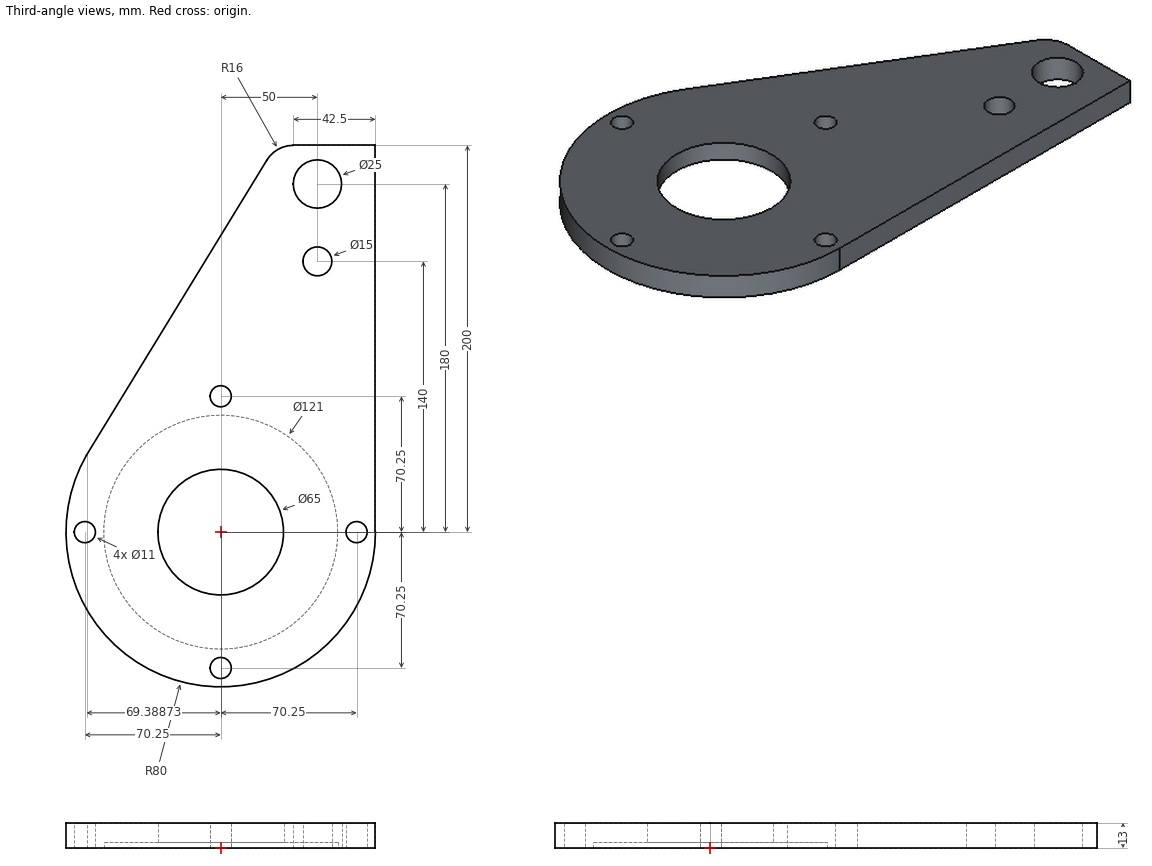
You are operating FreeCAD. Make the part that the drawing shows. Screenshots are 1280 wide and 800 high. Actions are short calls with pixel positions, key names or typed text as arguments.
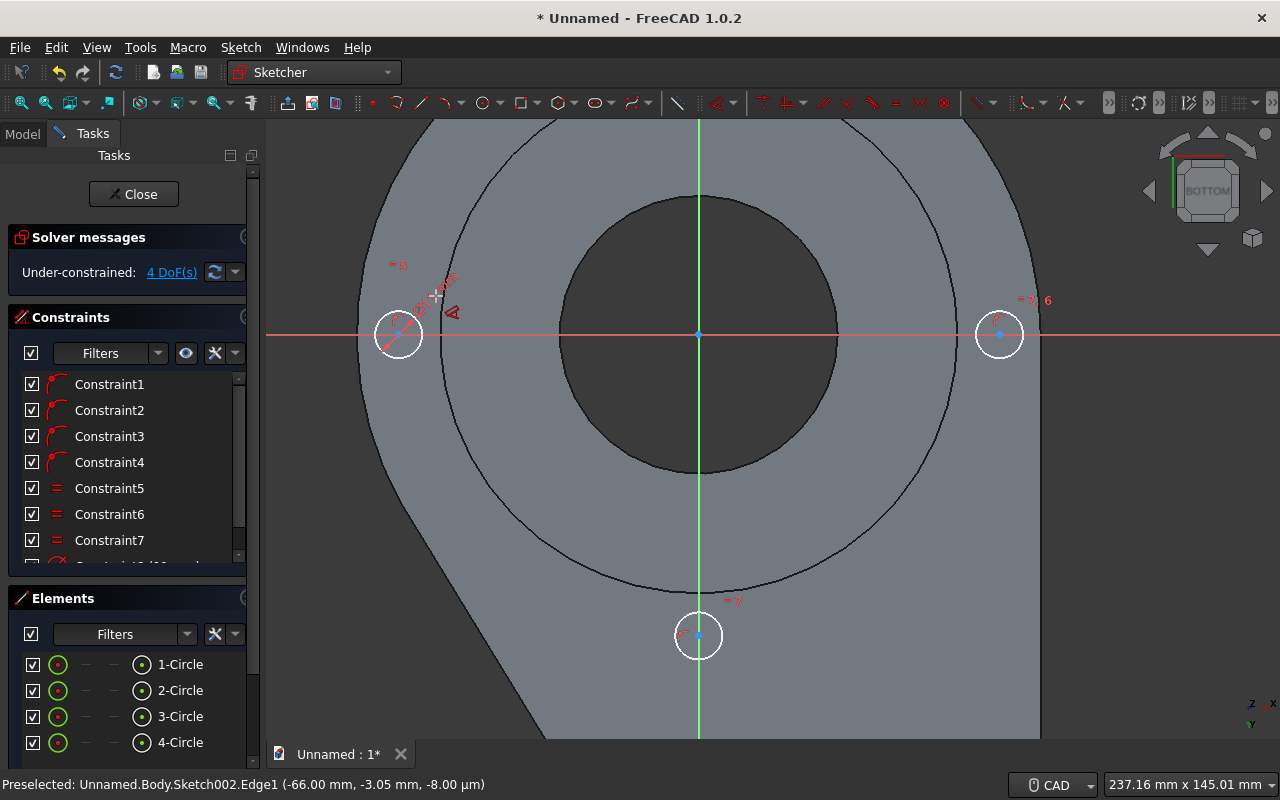
click(399, 335)
click(549, 369)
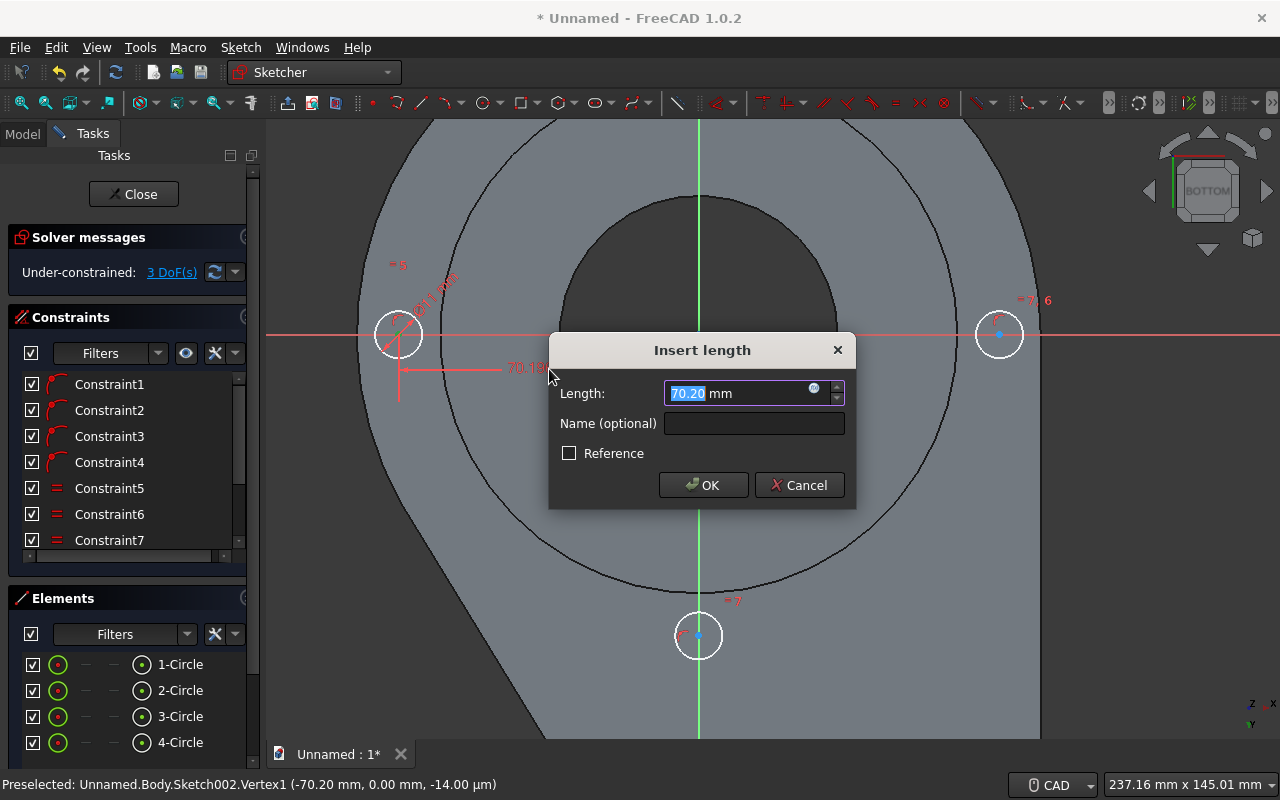
text(70.25)
key(Return)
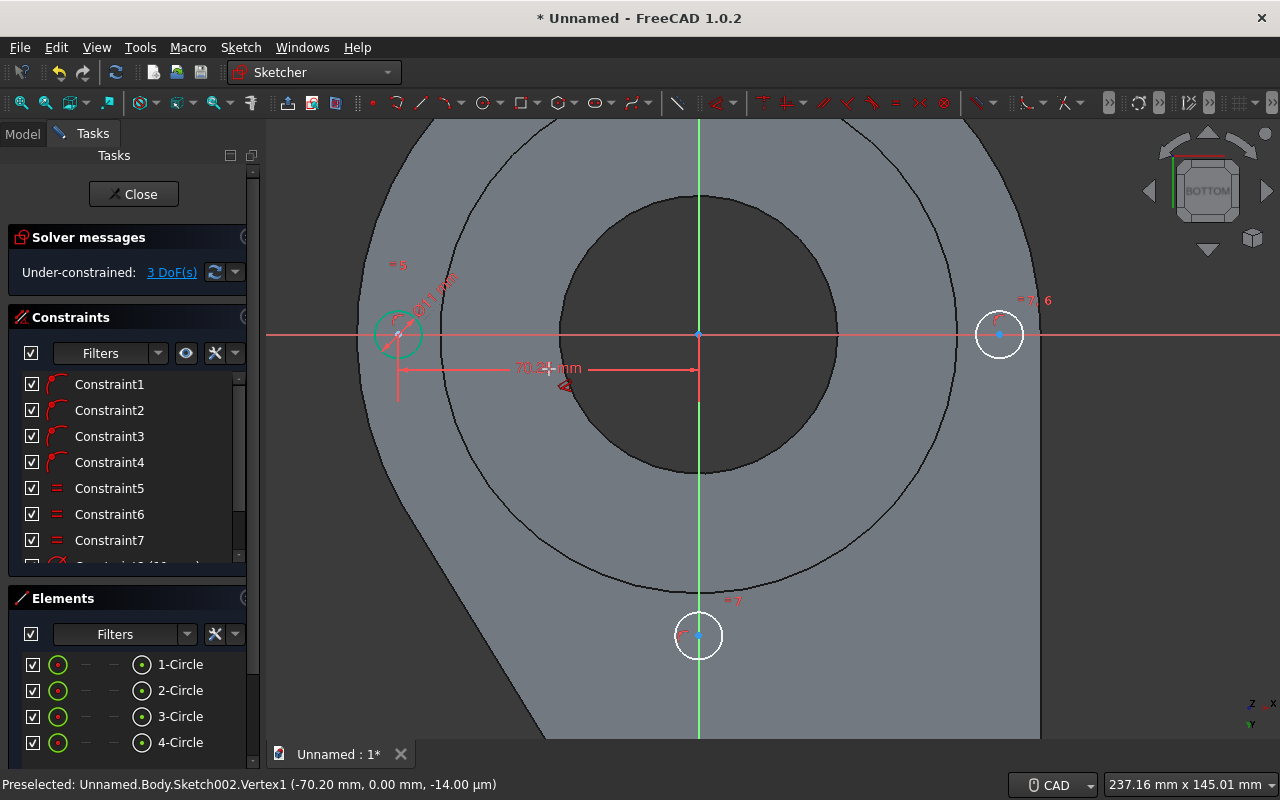
scroll(716, 621, down, 2)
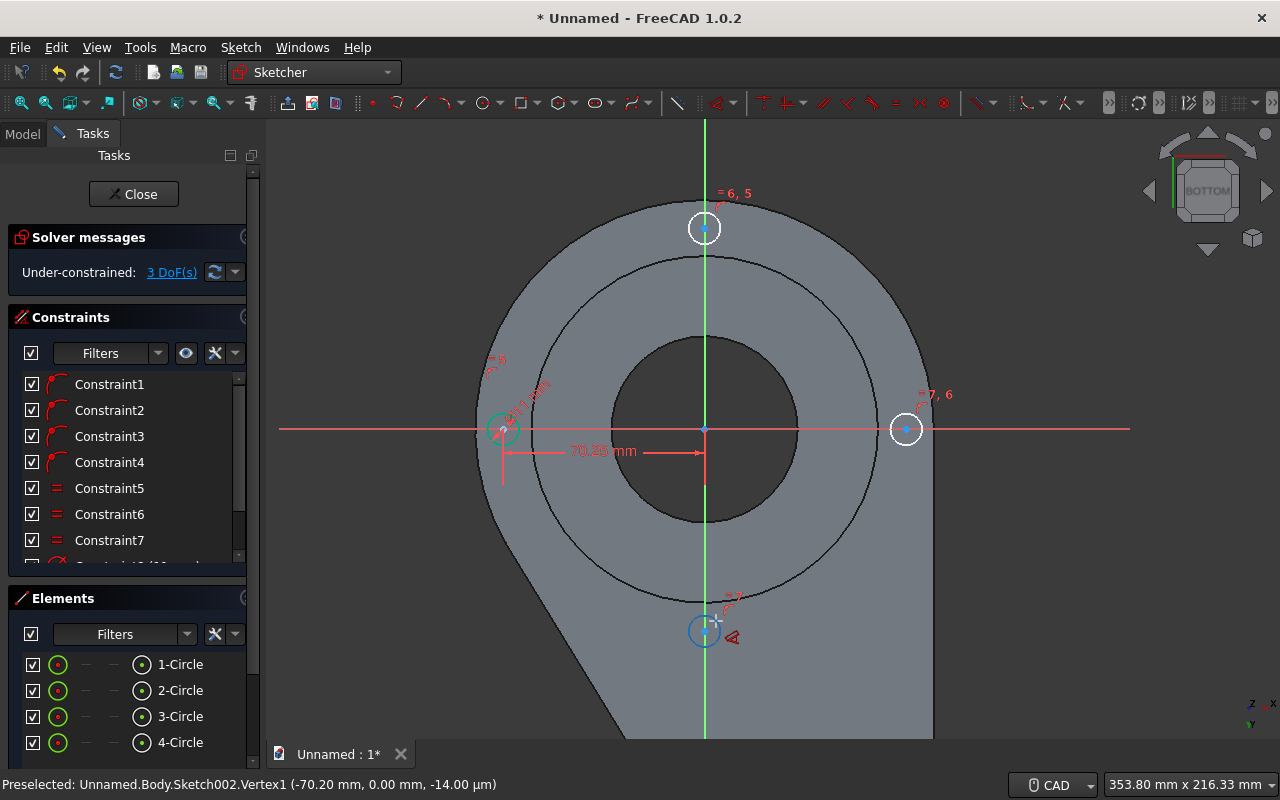
click(705, 228)
click(739, 329)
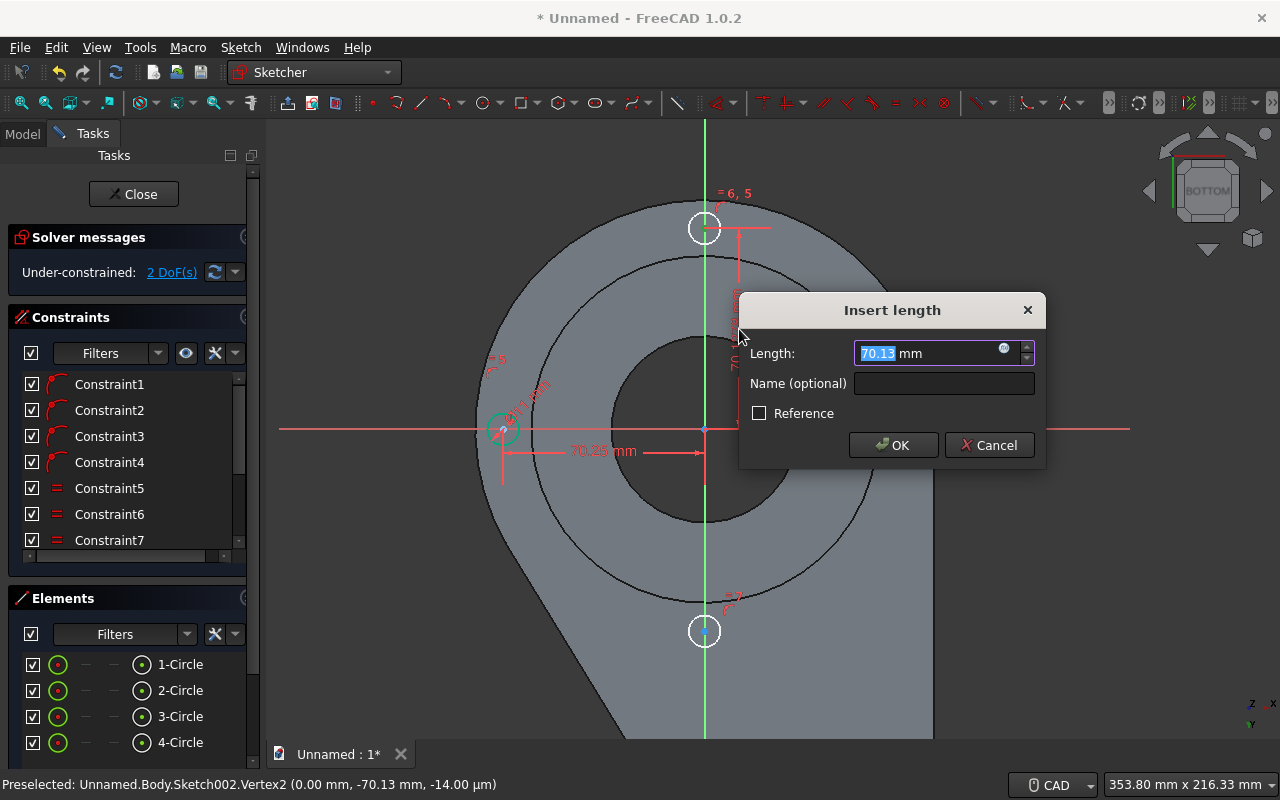
text(70.25)
key(Return)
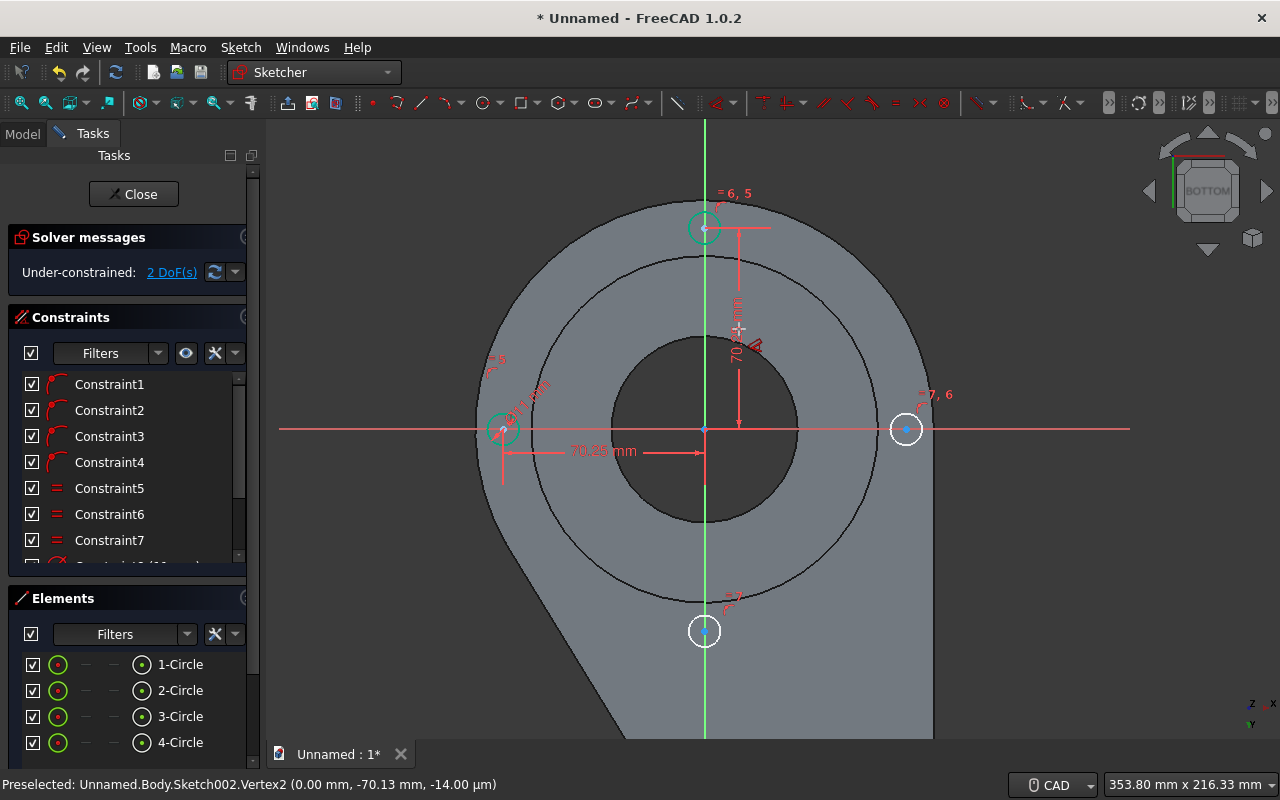
click(906, 429)
click(805, 463)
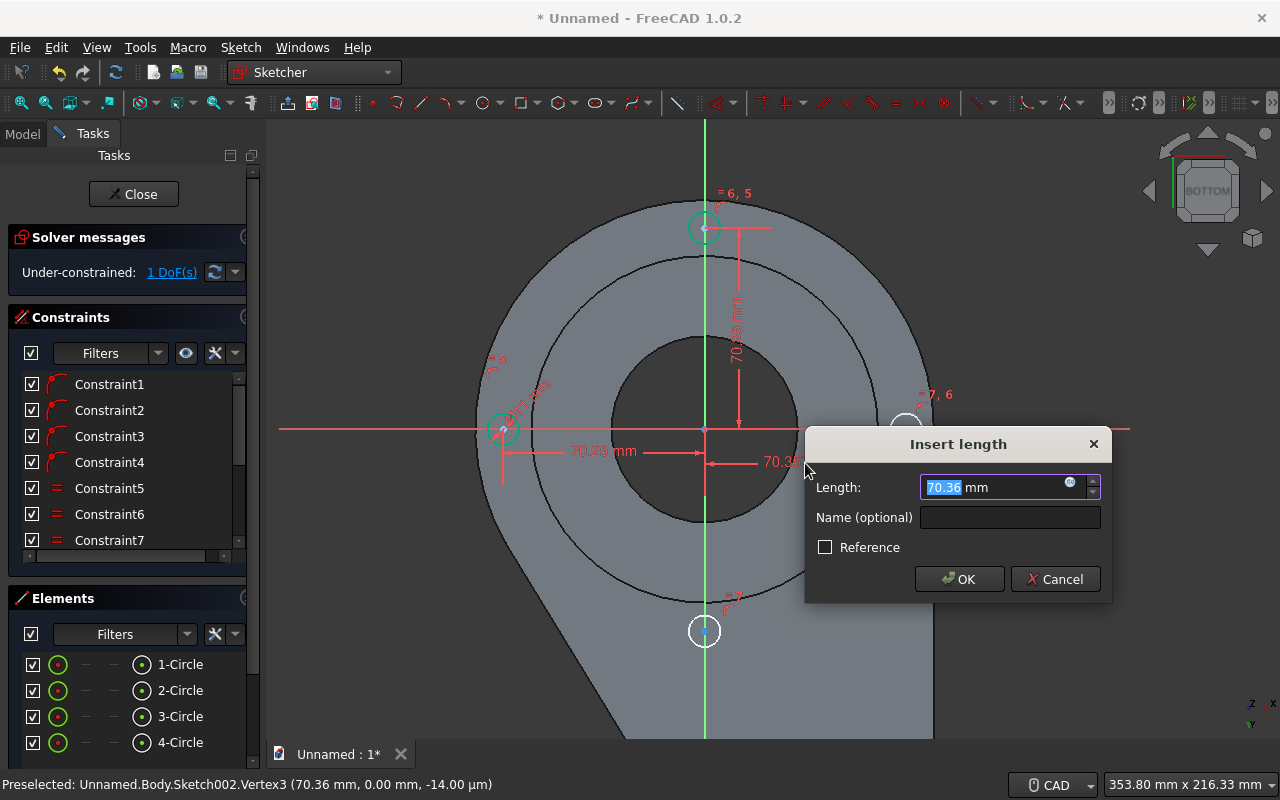
text(70.25)
key(Return)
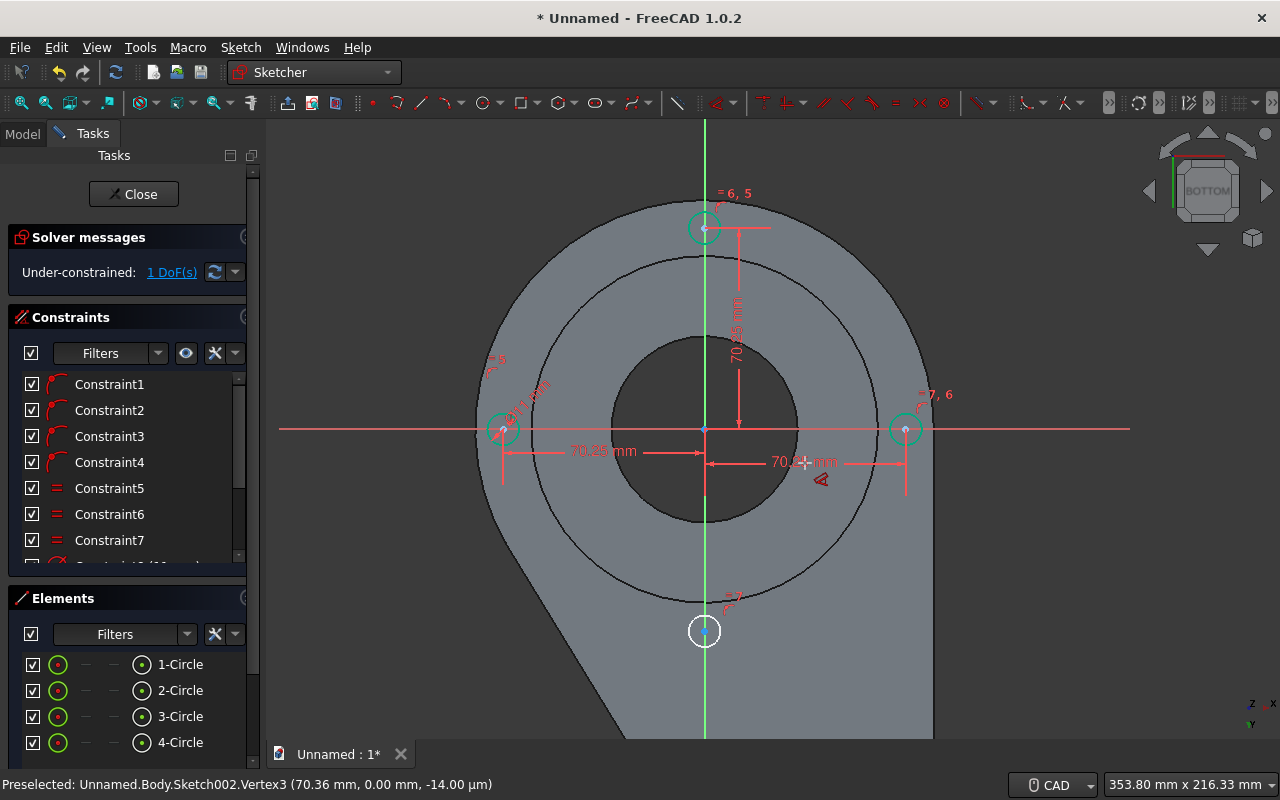
click(705, 631)
click(739, 530)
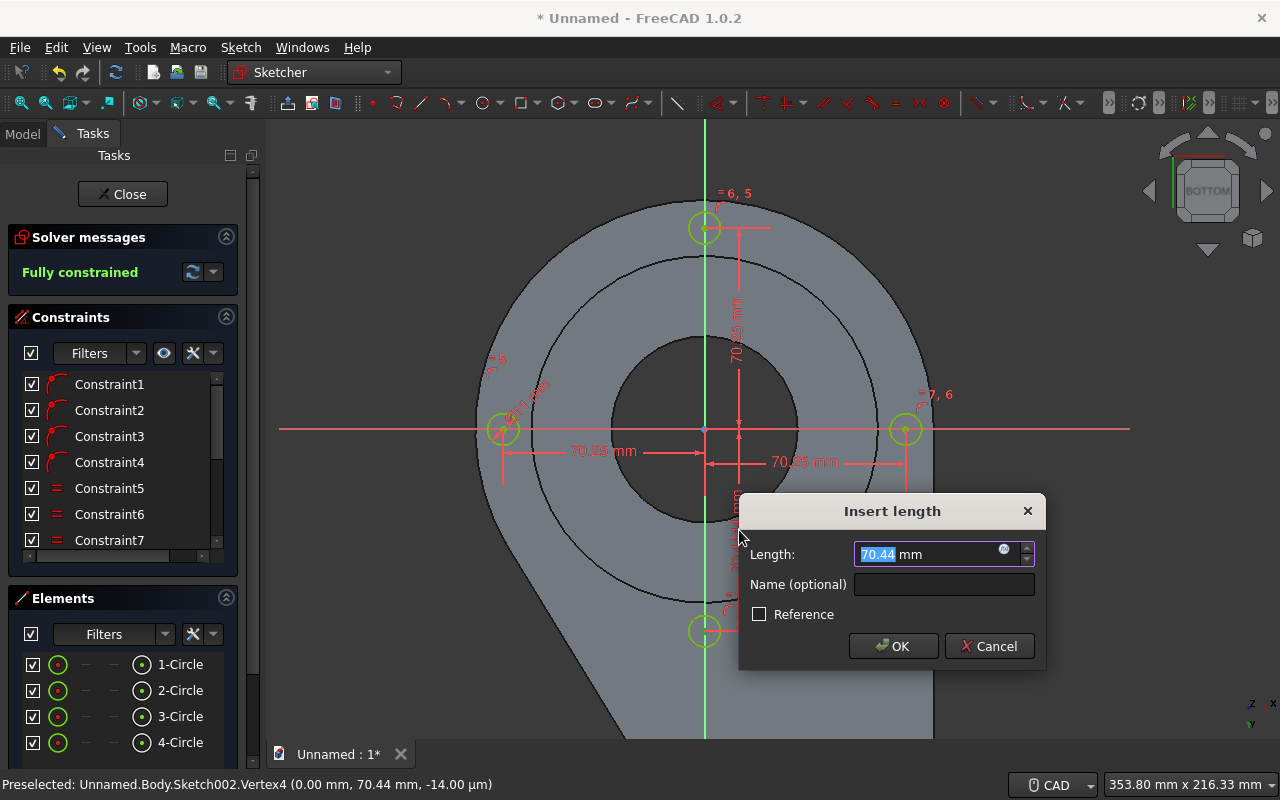
text(70.25)
key(Return)
key(Escape)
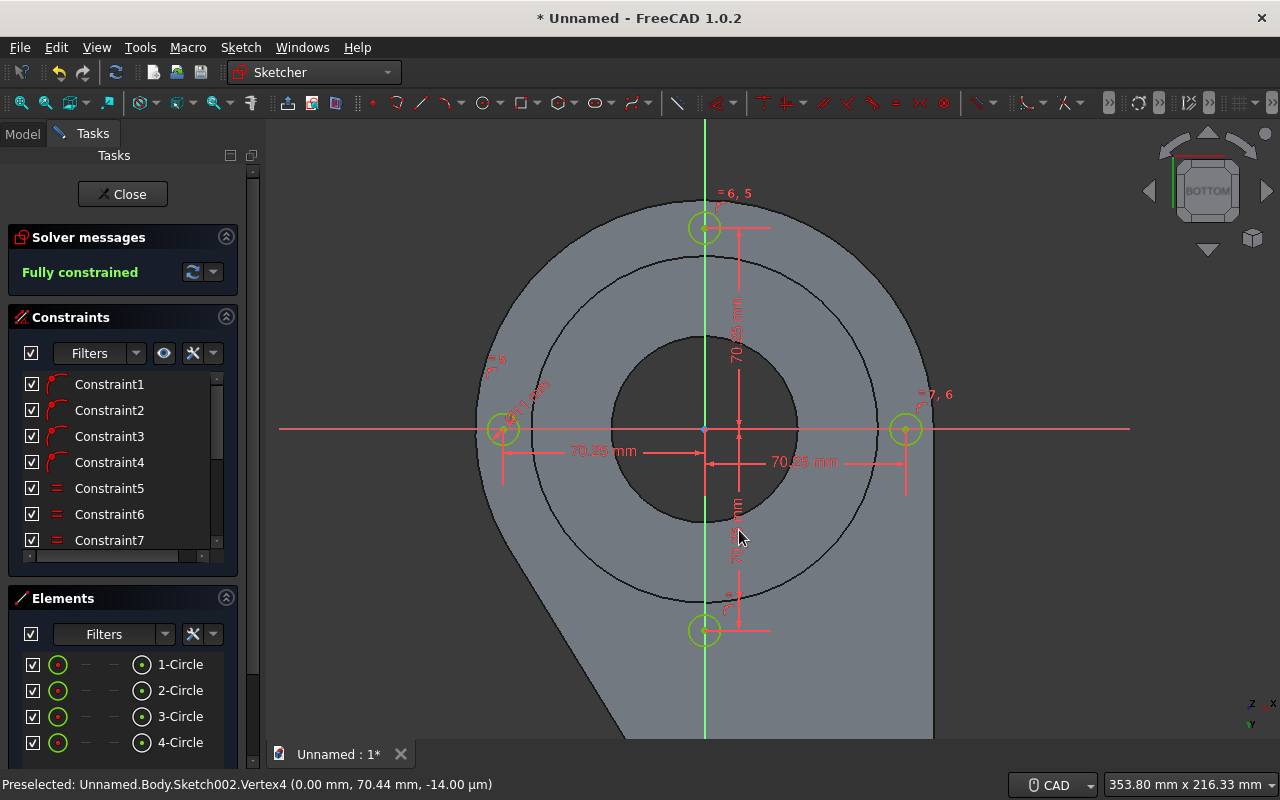
click(123, 194)